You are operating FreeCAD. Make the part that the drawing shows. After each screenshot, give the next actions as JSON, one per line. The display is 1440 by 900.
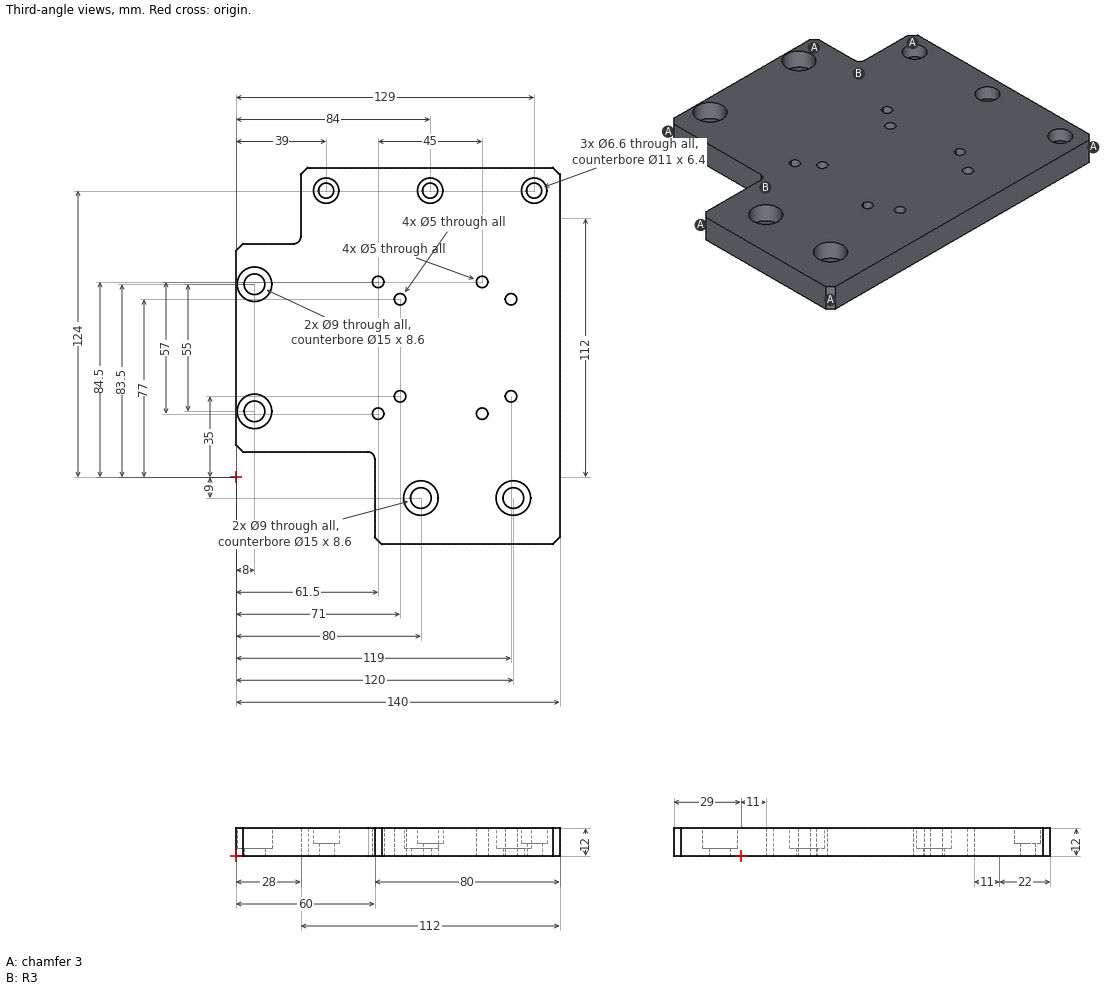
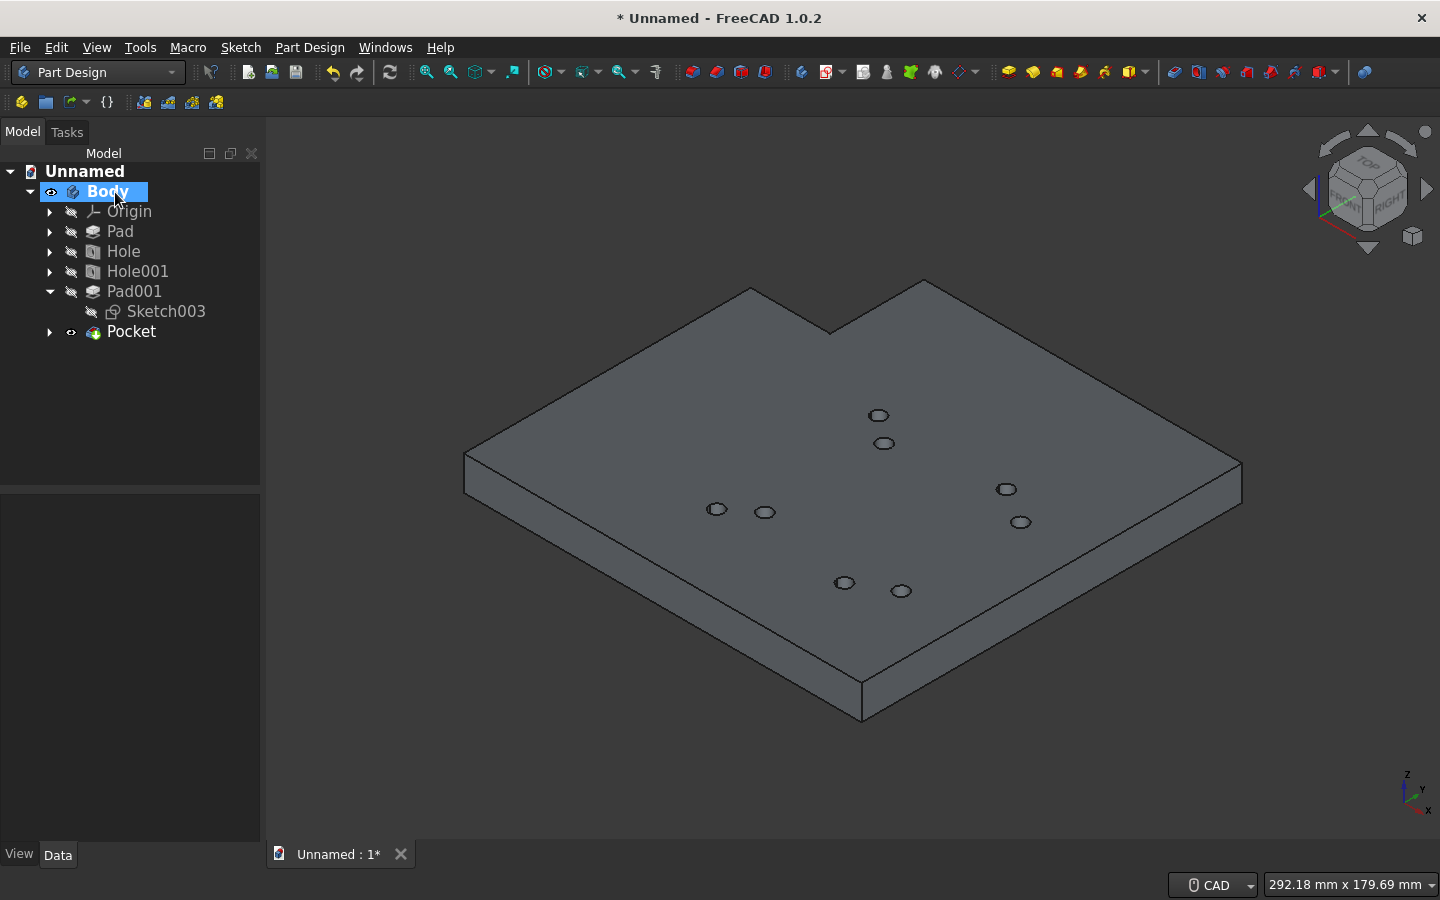
{"action": "left_click", "coordinate": [833, 685]}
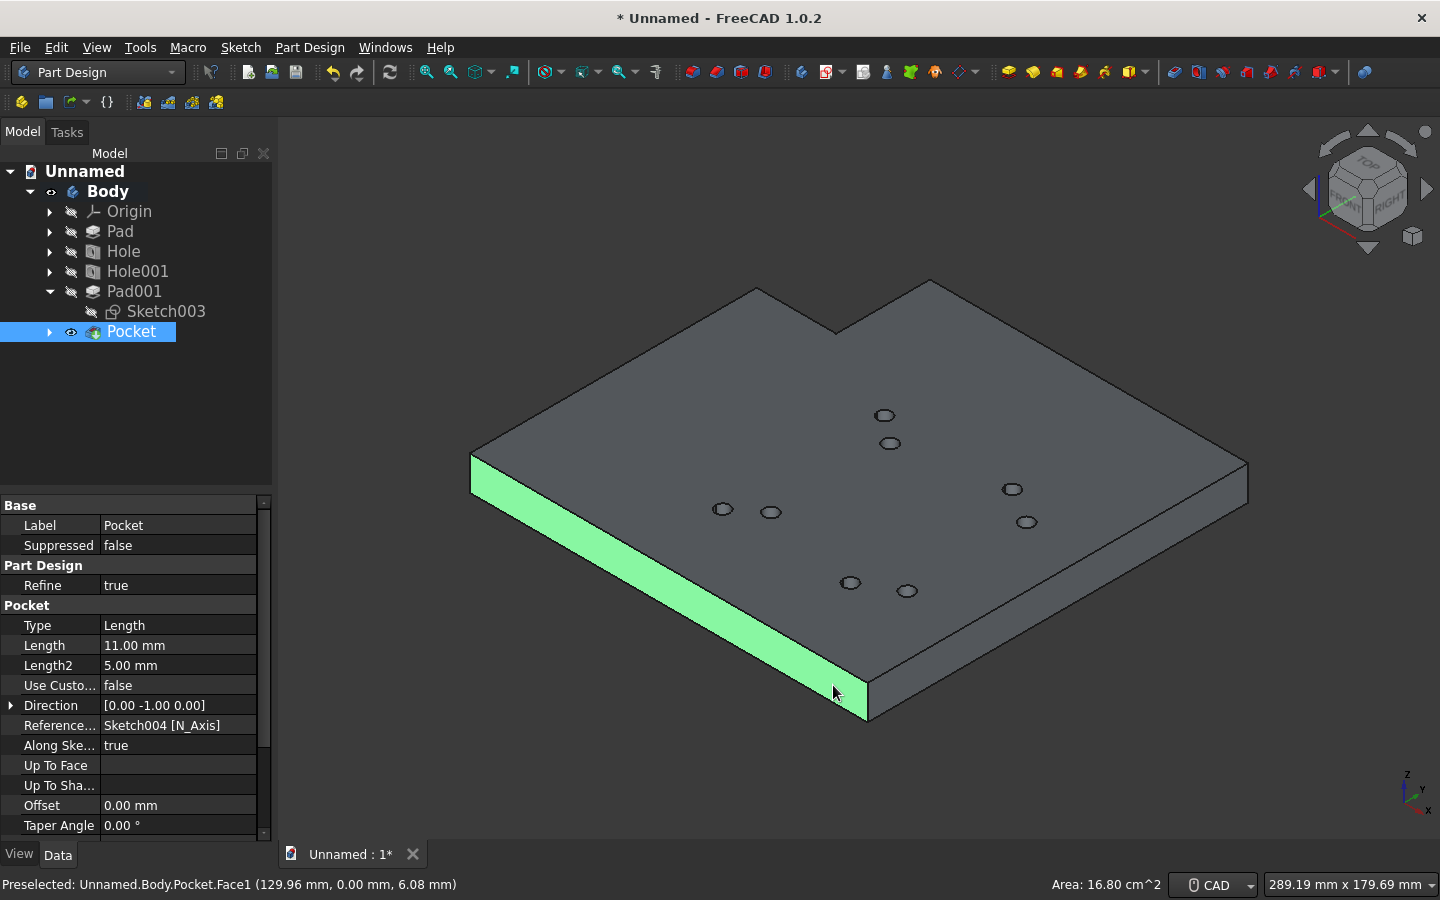
{"action": "left_click", "coordinate": [826, 72]}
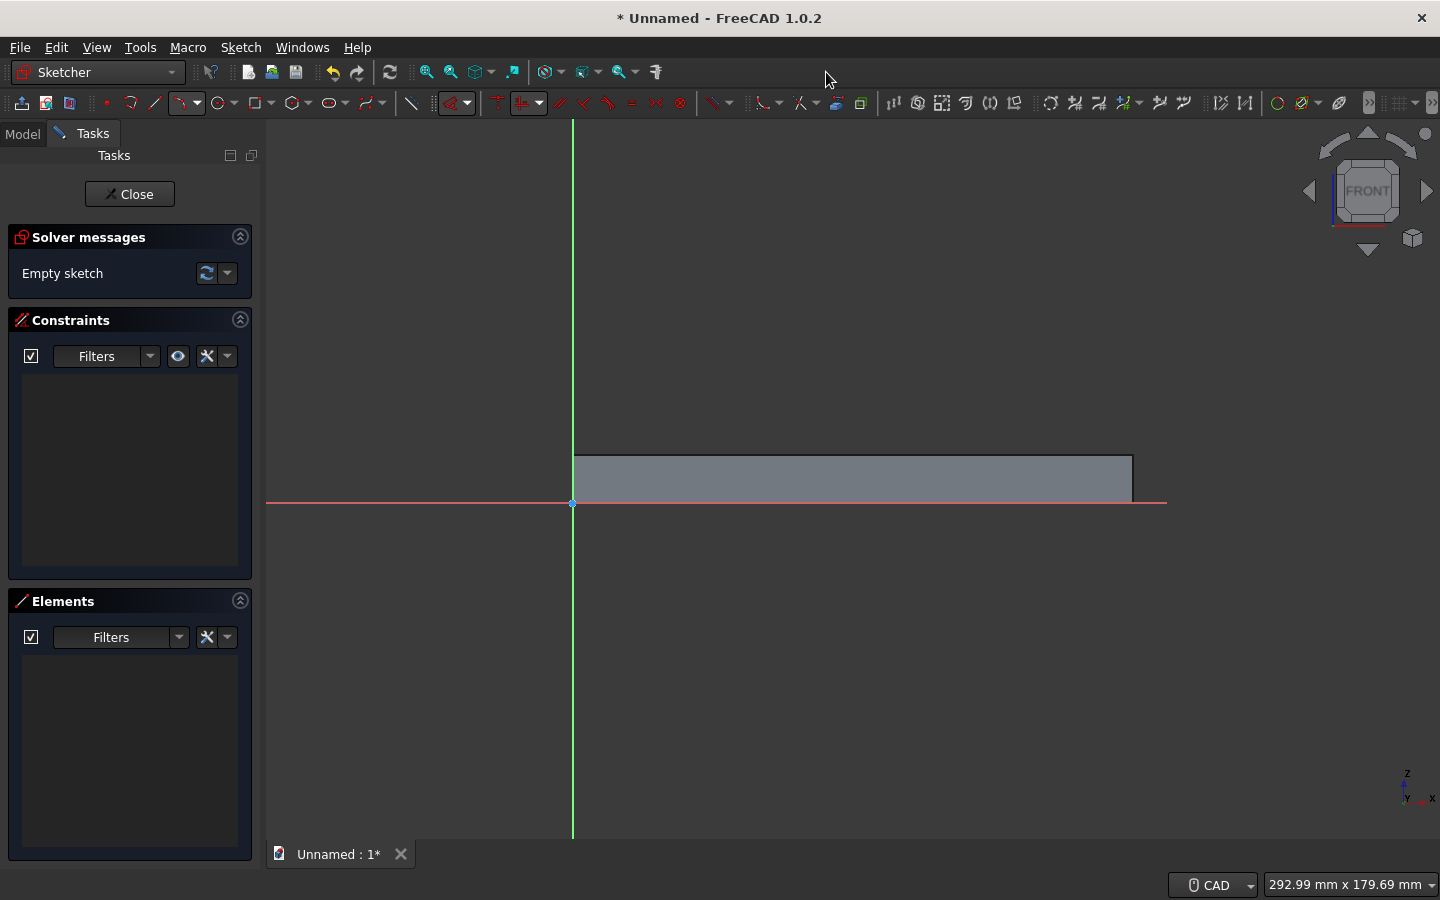
{"action": "scroll", "coordinate": [639, 479], "scroll_direction": "up", "scroll_amount": 5}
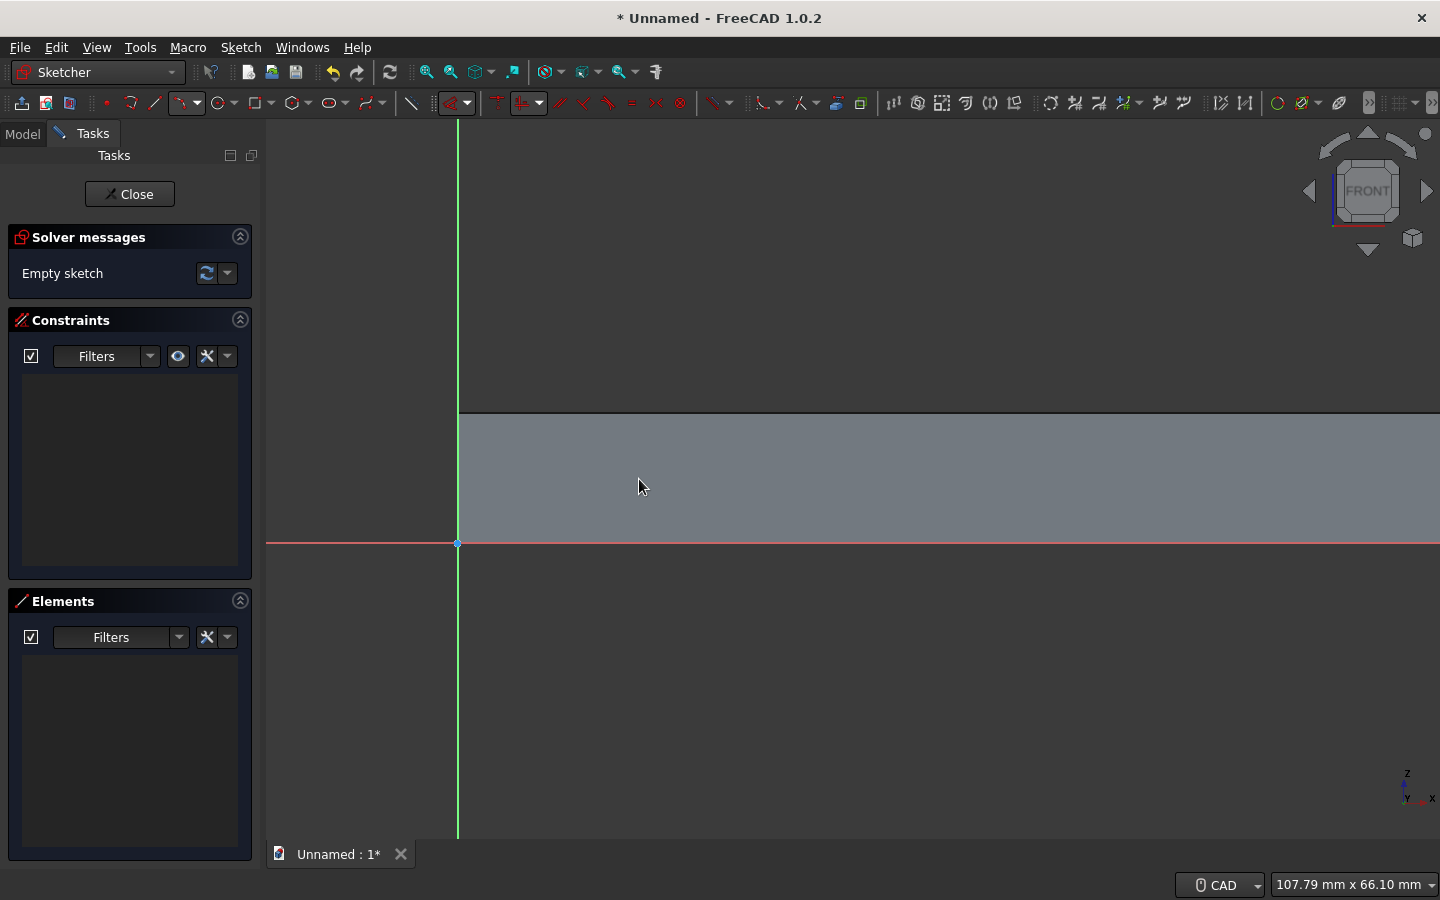
{"action": "left_click", "coordinate": [256, 104]}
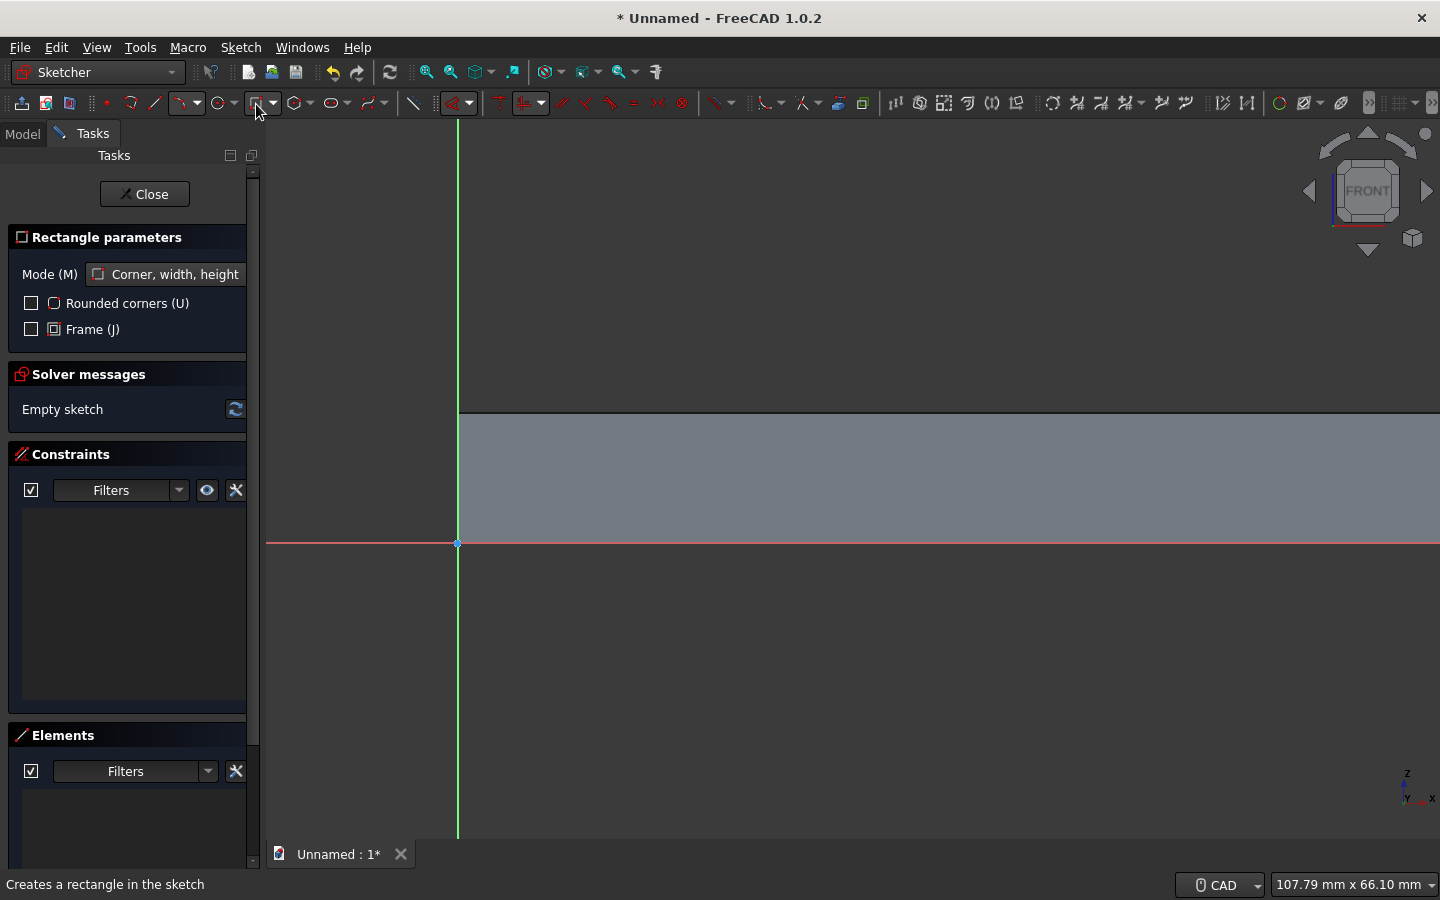
{"action": "left_click", "coordinate": [458, 543]}
{"action": "mouse_move", "coordinate": [1111, 413]}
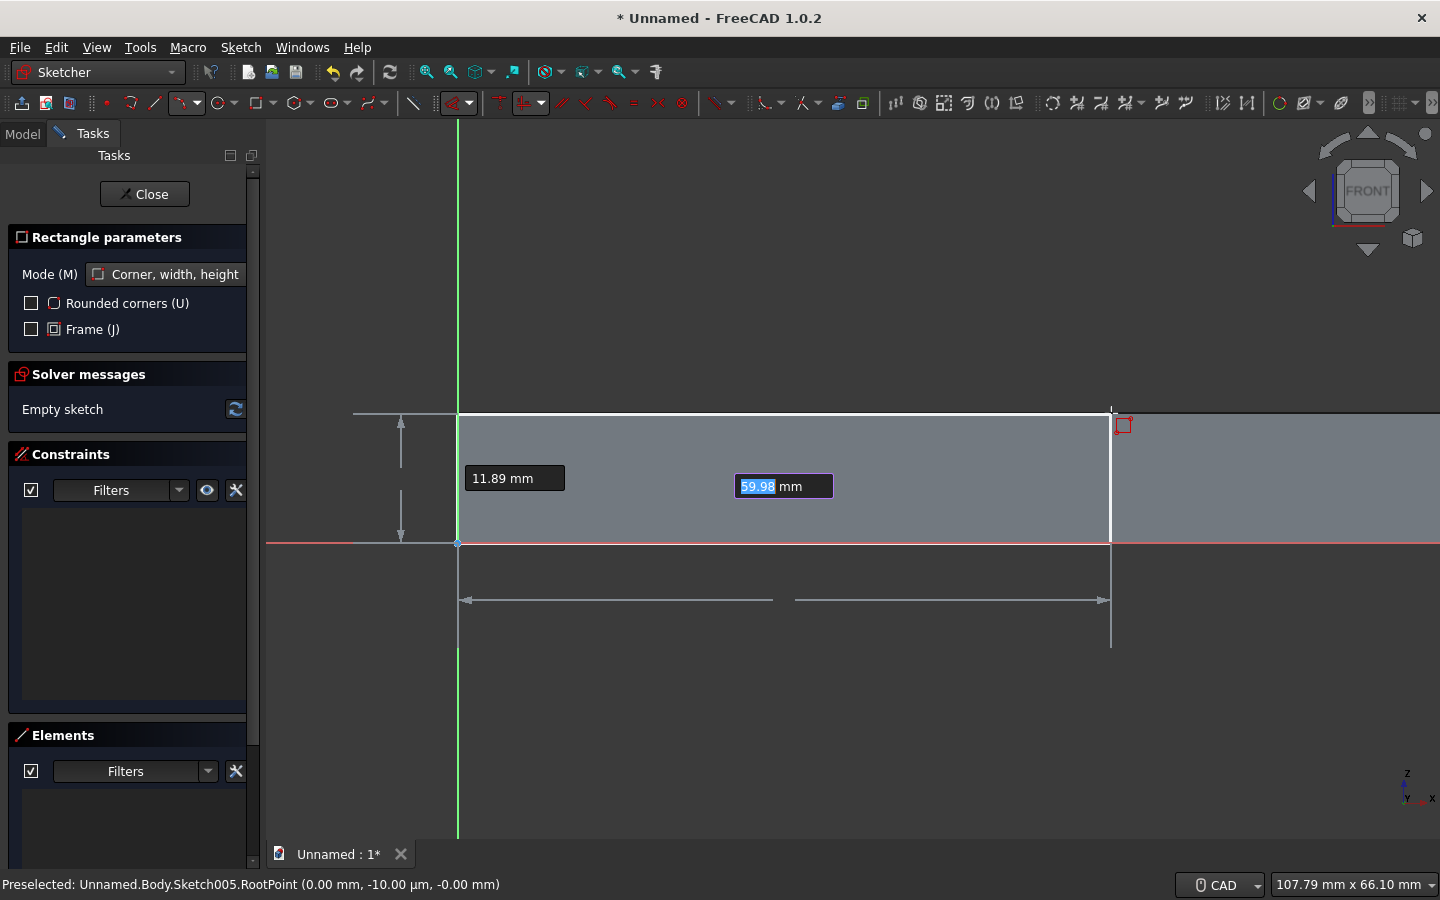
{"action": "type", "text": "60"}
{"action": "key", "text": "Tab"}
{"action": "type", "text": "12"}
{"action": "key", "text": "Return"}
{"action": "key", "text": "Escape"}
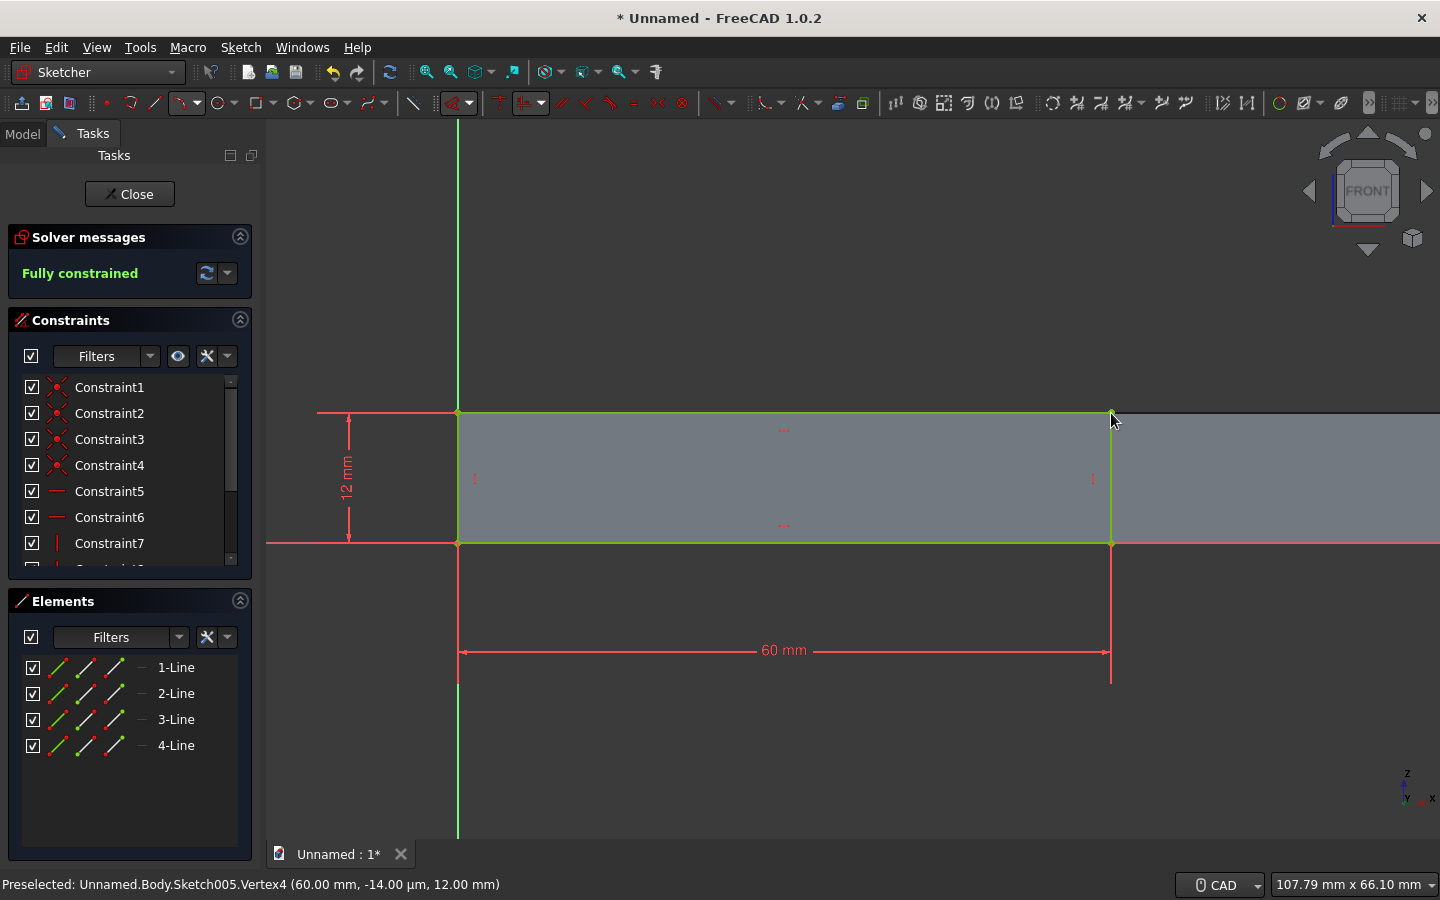
{"action": "left_click", "coordinate": [130, 194]}